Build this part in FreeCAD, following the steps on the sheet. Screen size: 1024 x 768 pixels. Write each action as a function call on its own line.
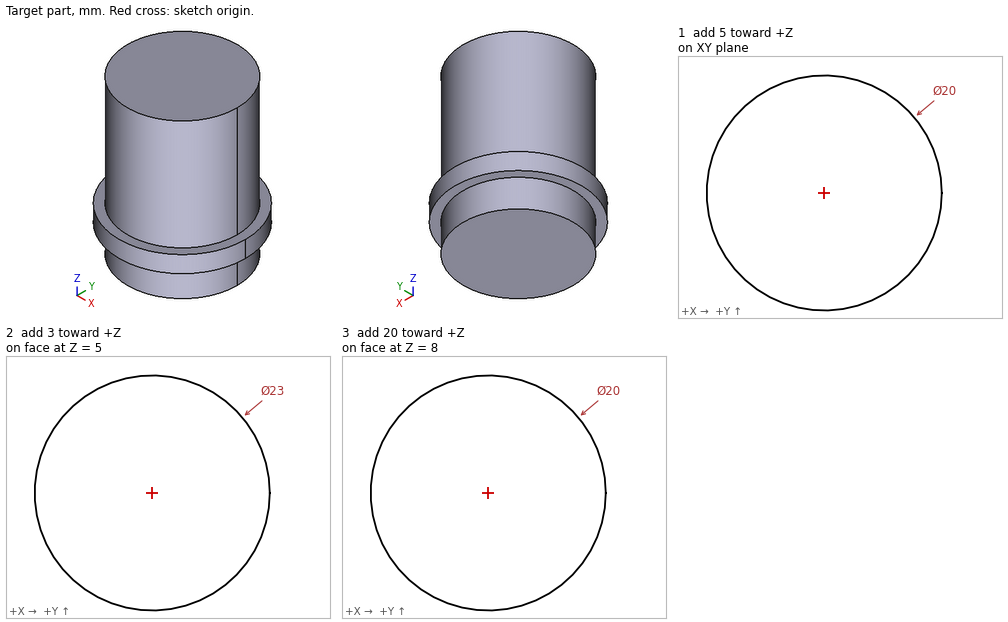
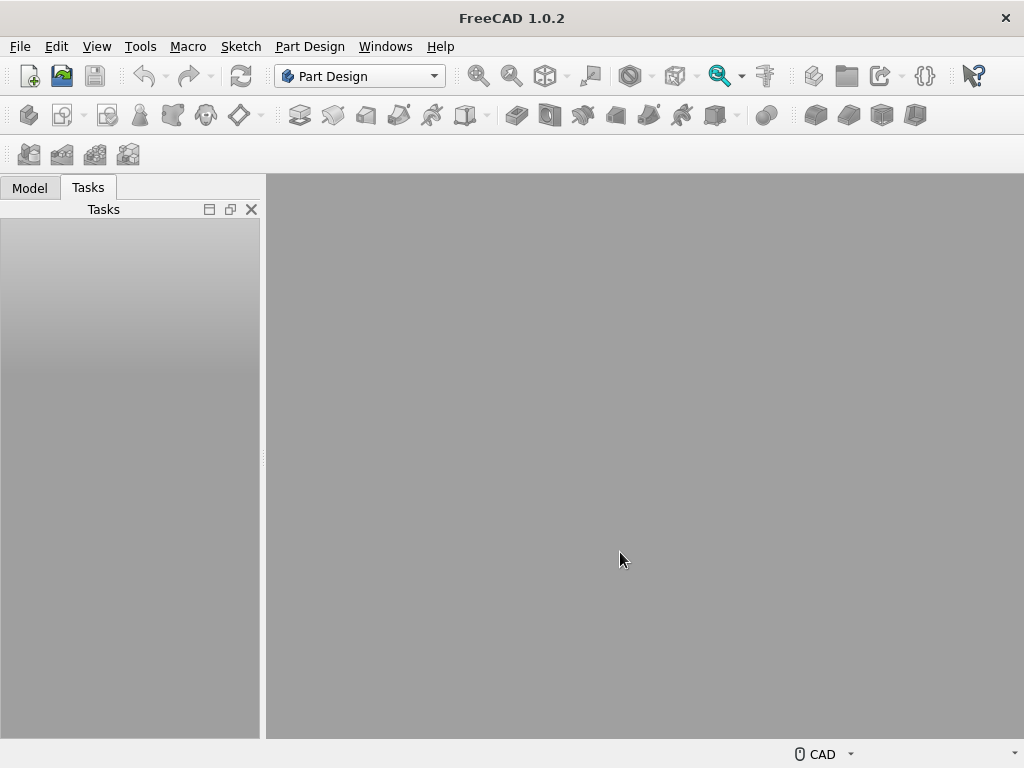
click(29, 76)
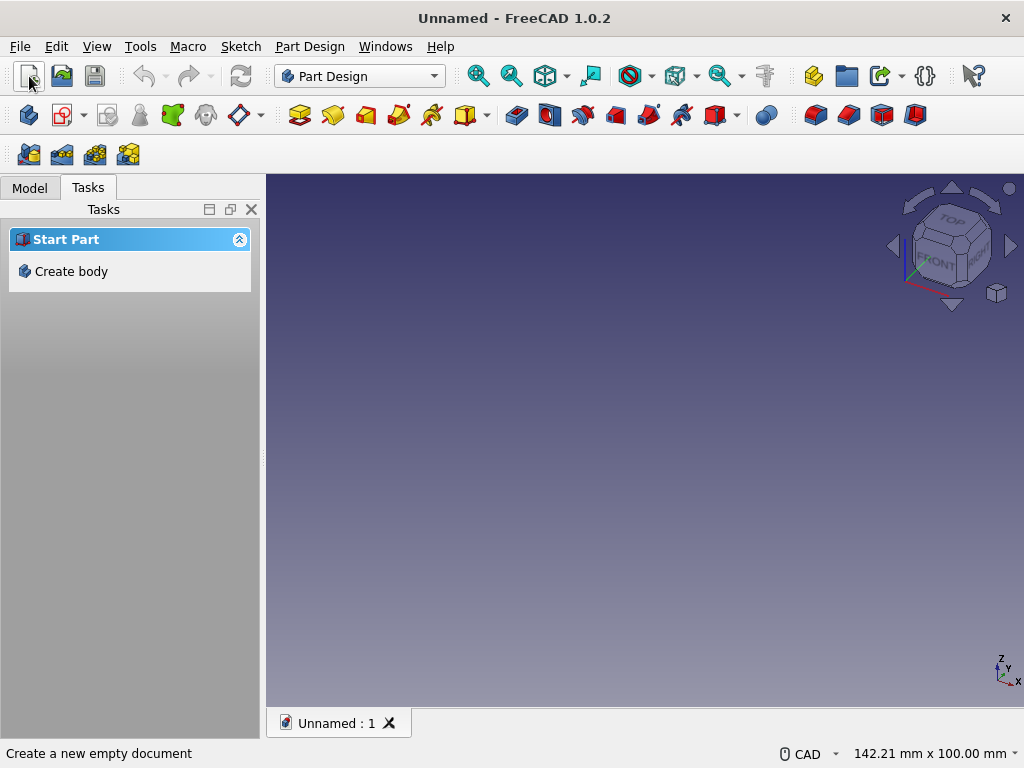
click(62, 116)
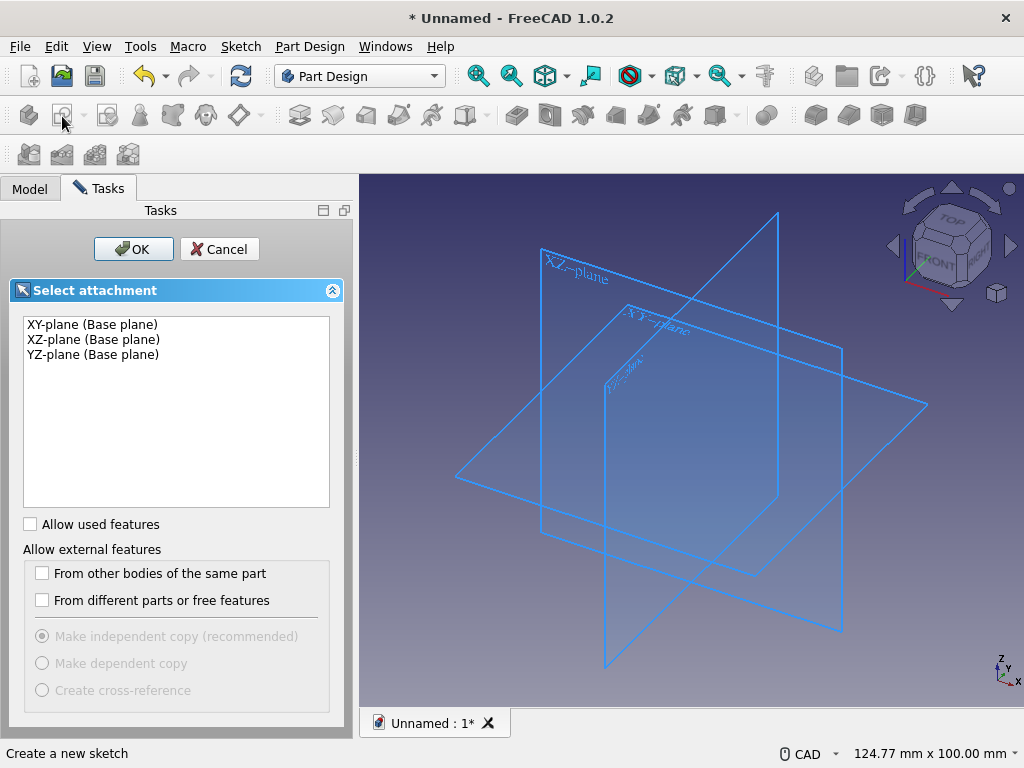
click(84, 324)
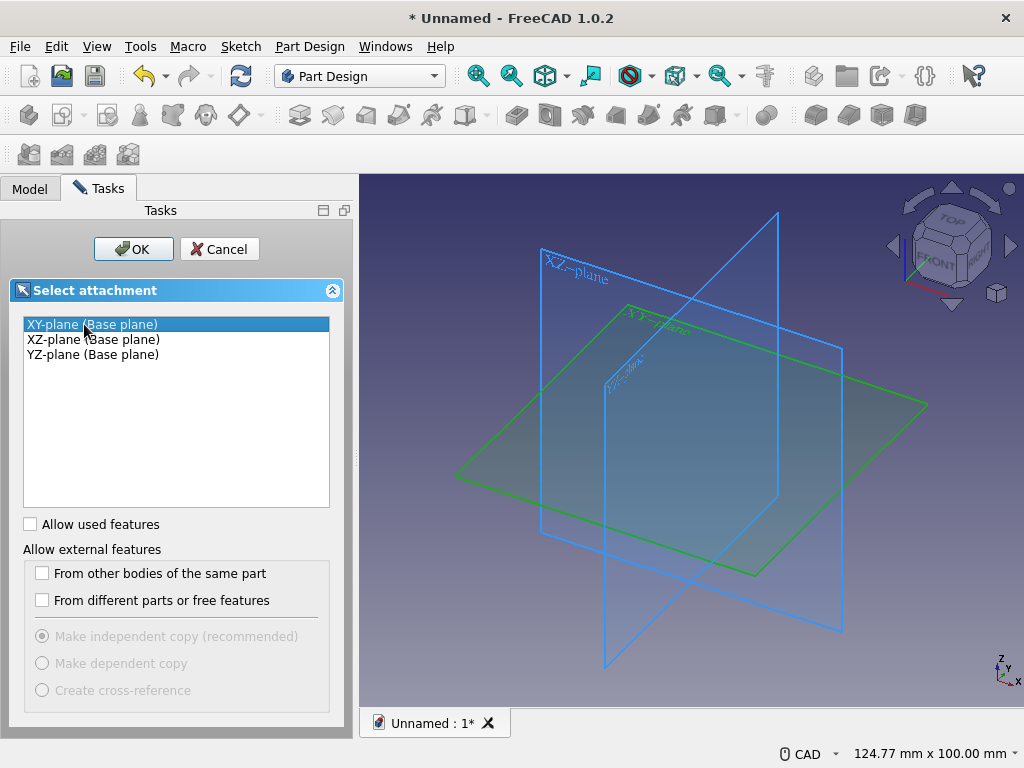
click(134, 249)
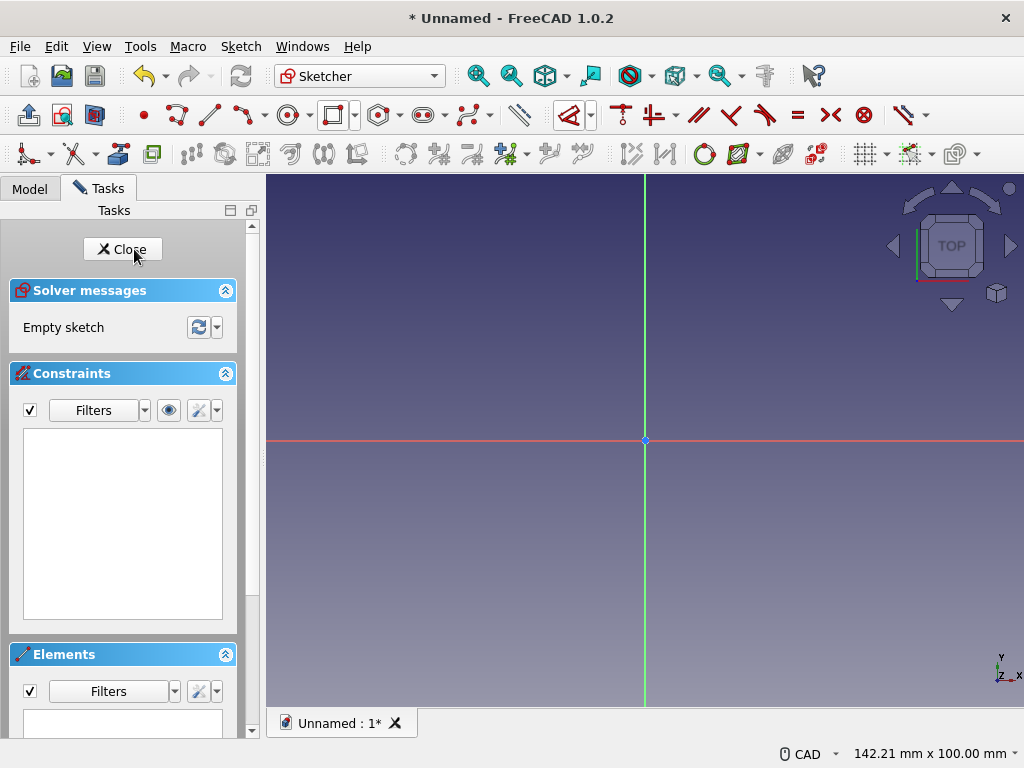
scroll(675, 440, up, 6)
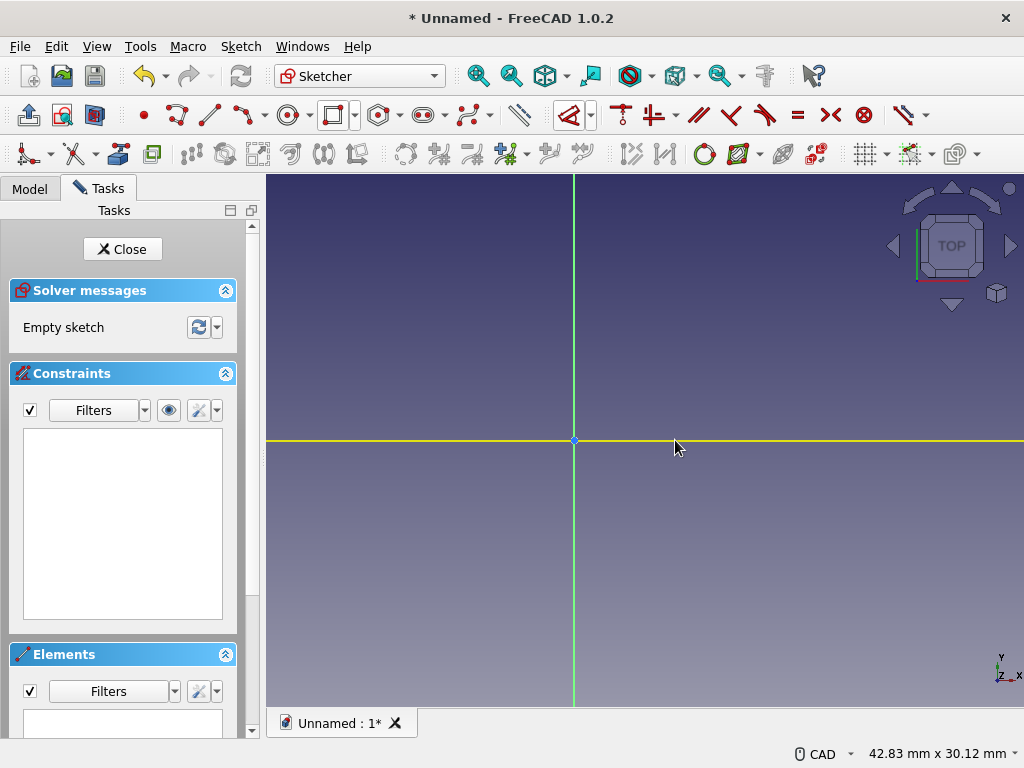
click(288, 116)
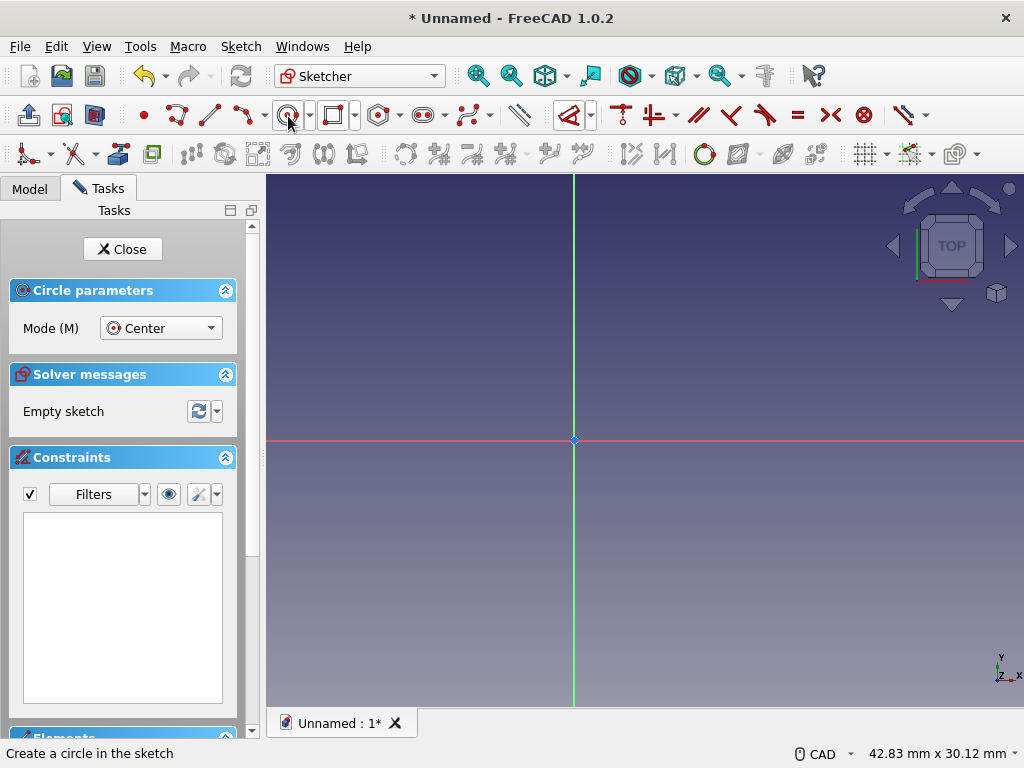
click(574, 440)
click(699, 315)
key(Escape)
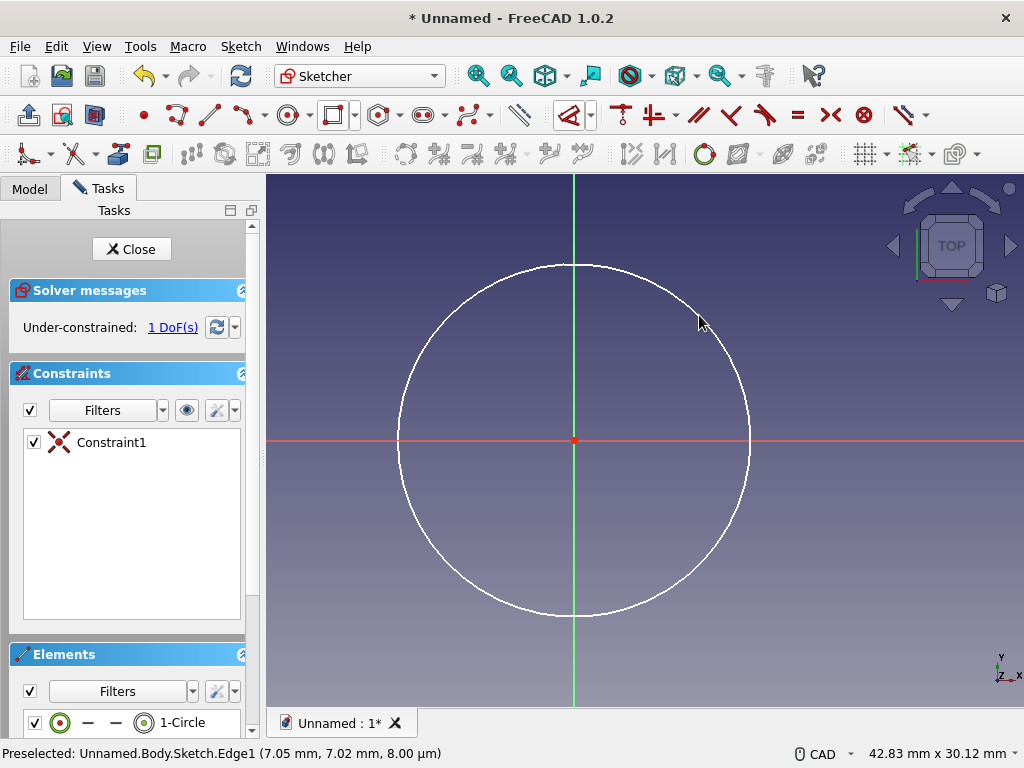
key(d)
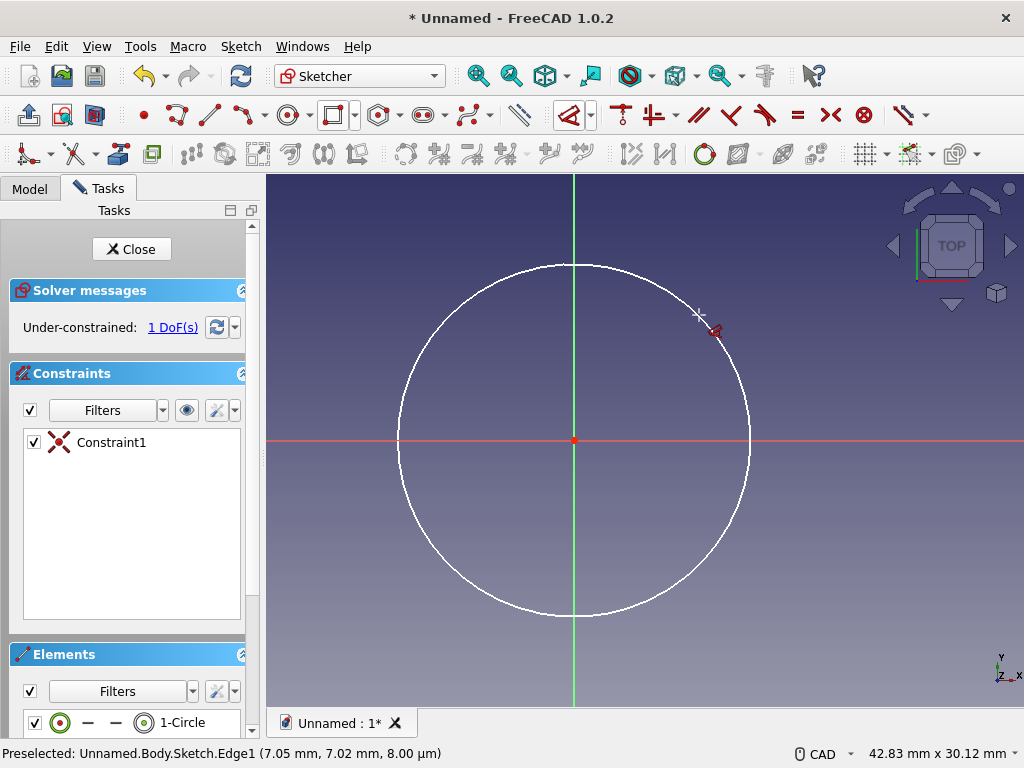
click(698, 315)
click(720, 292)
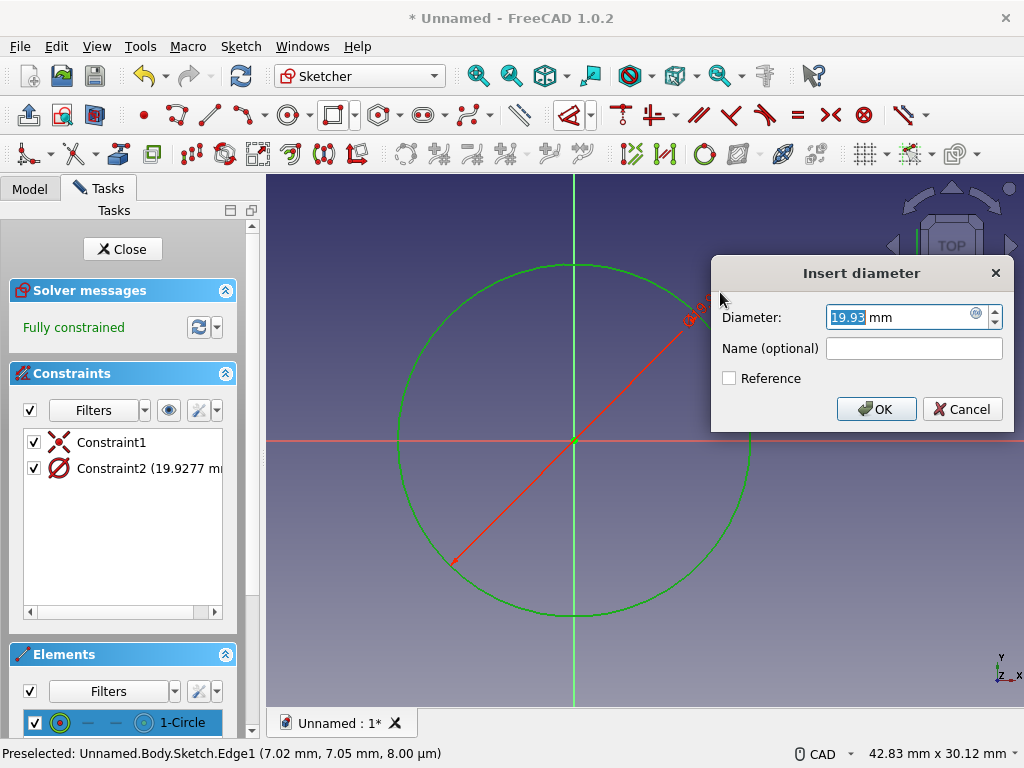
text(20)
key(Return)
key(Escape)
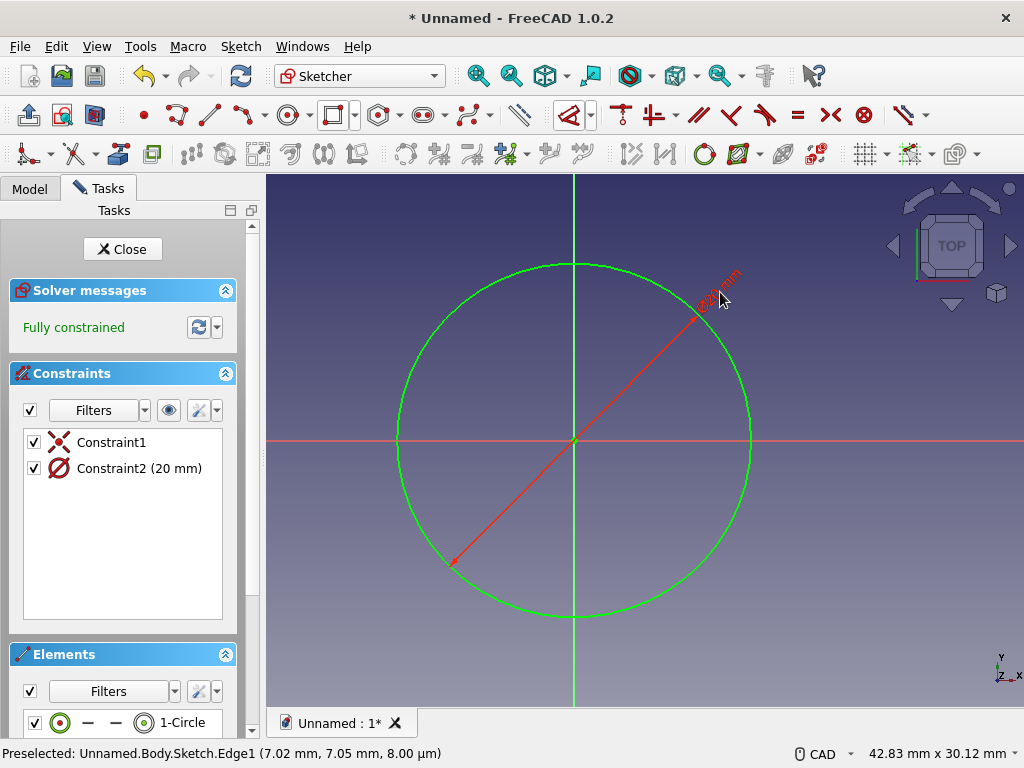
click(123, 249)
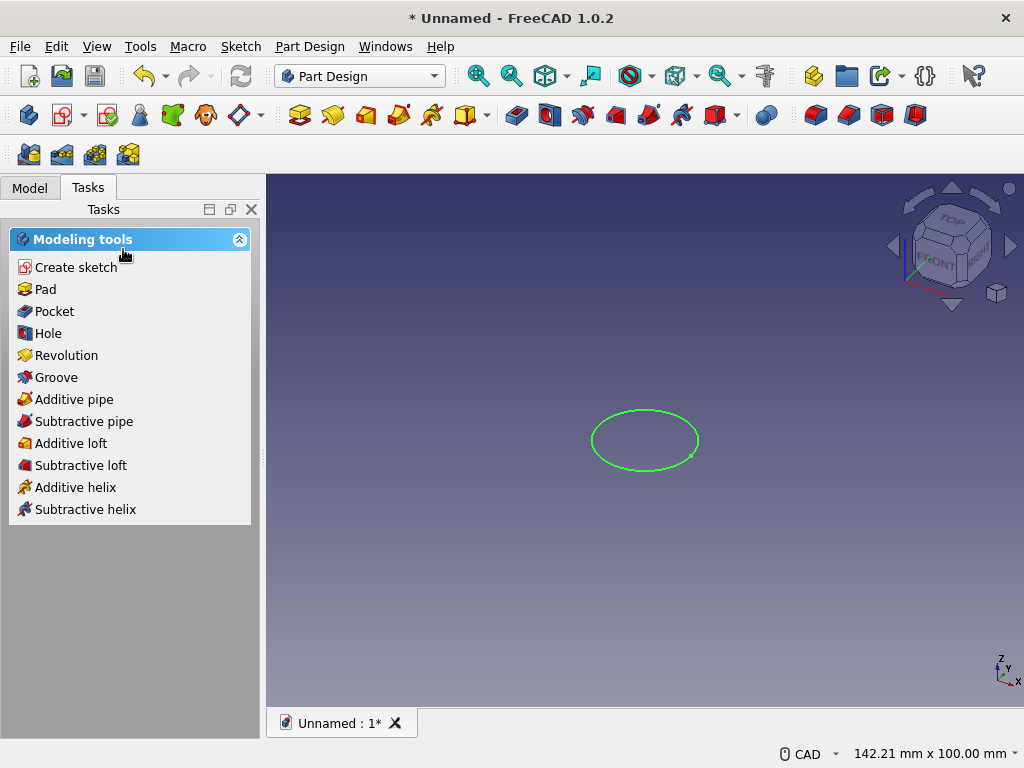
click(300, 116)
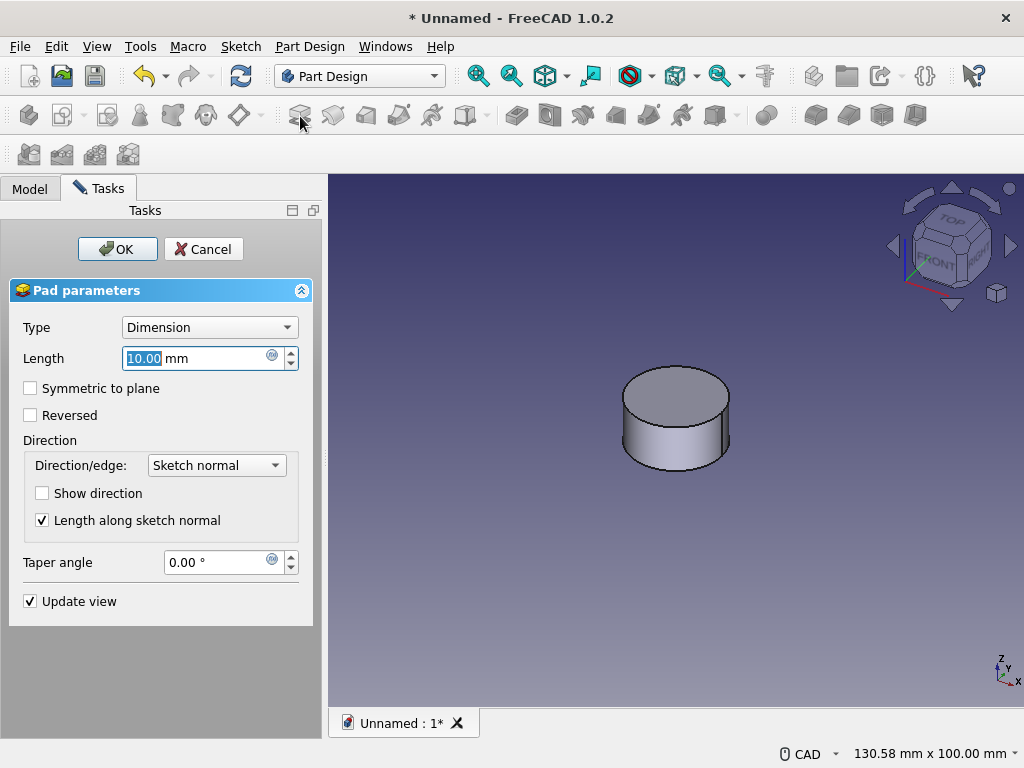
text(5)
key(Tab)